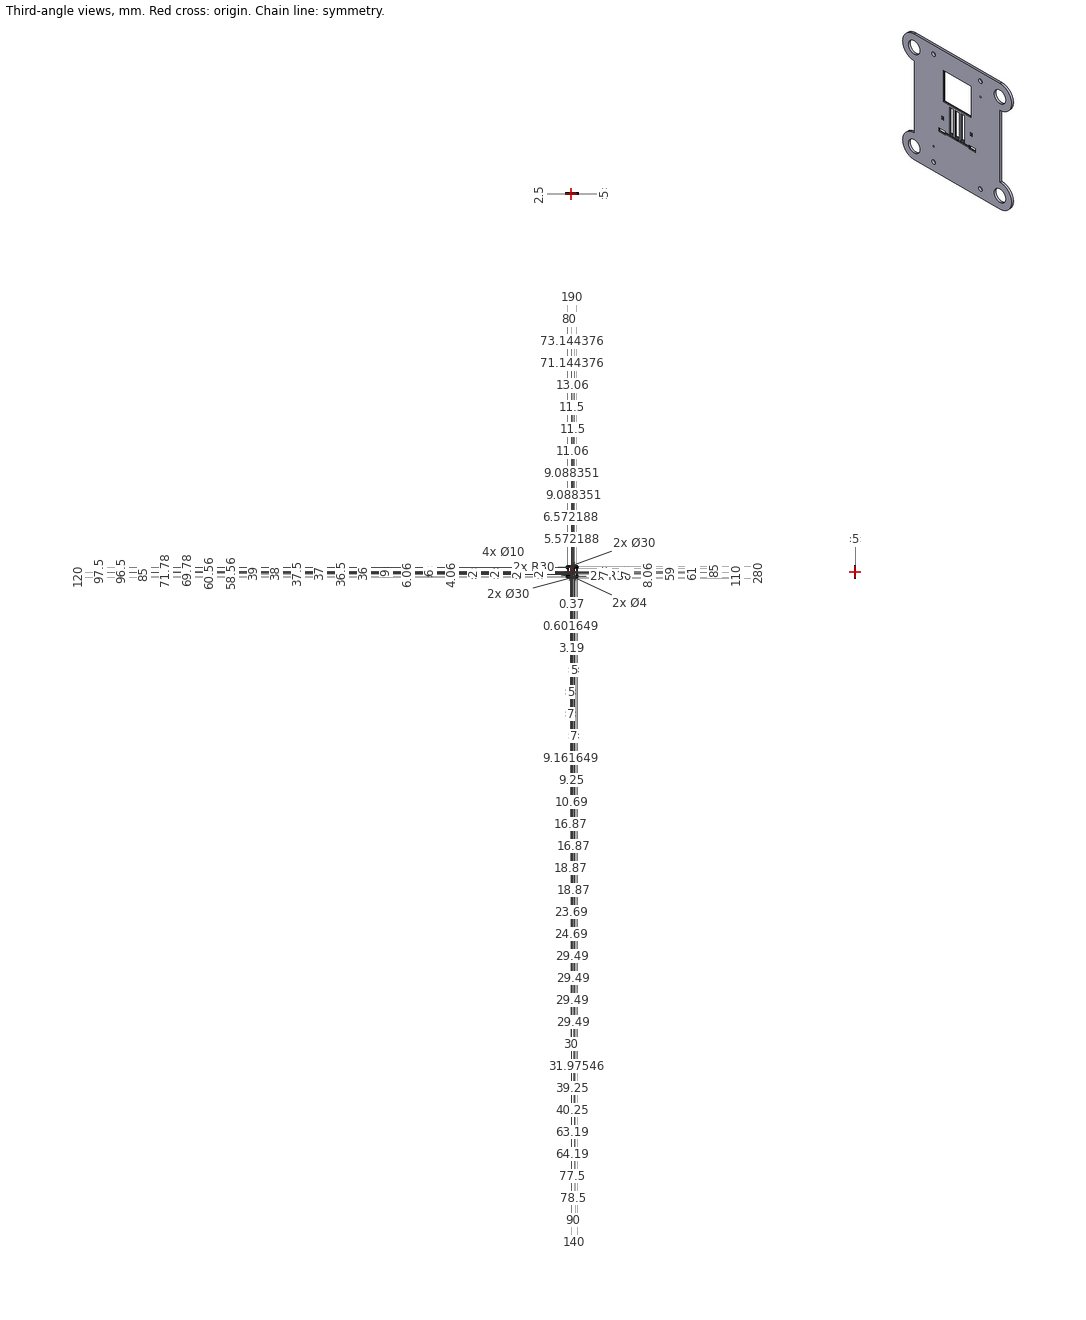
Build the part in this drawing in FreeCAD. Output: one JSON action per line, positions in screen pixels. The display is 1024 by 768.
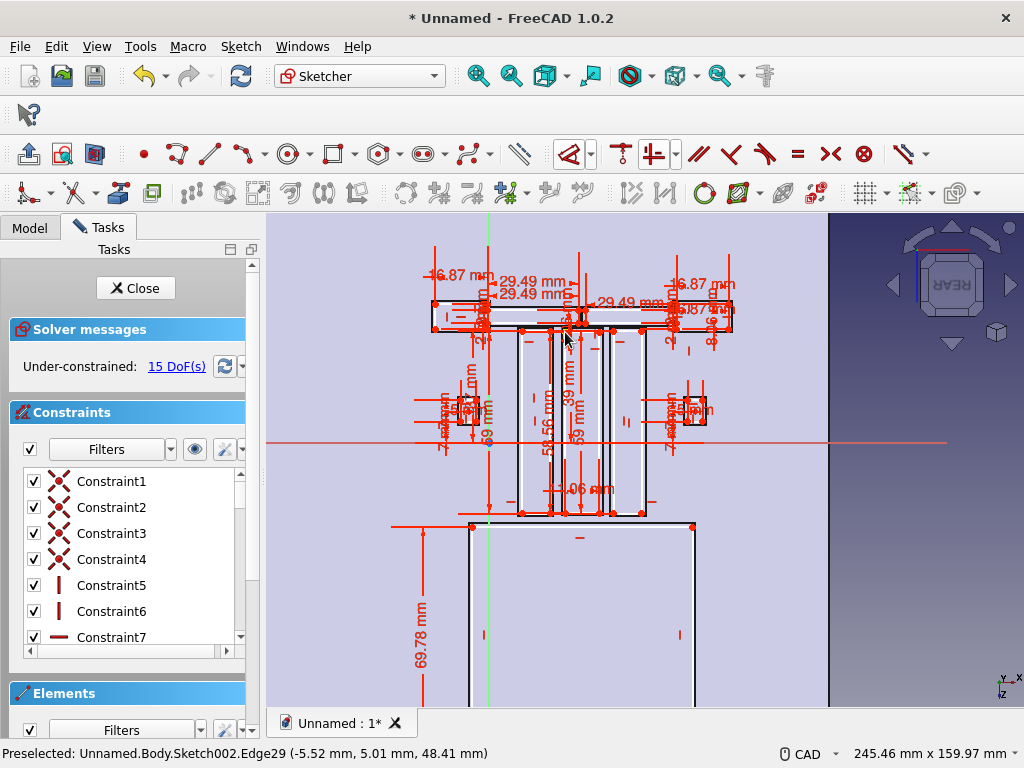
{"action": "left_click", "coordinate": [565, 332]}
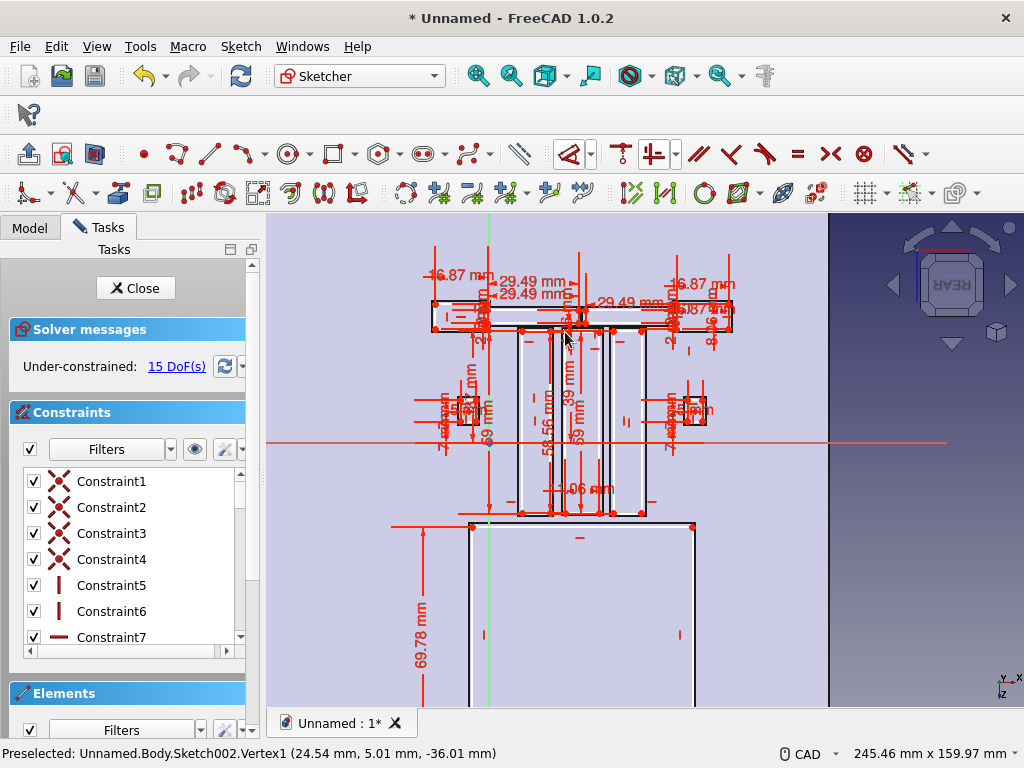
{"action": "key", "text": "i"}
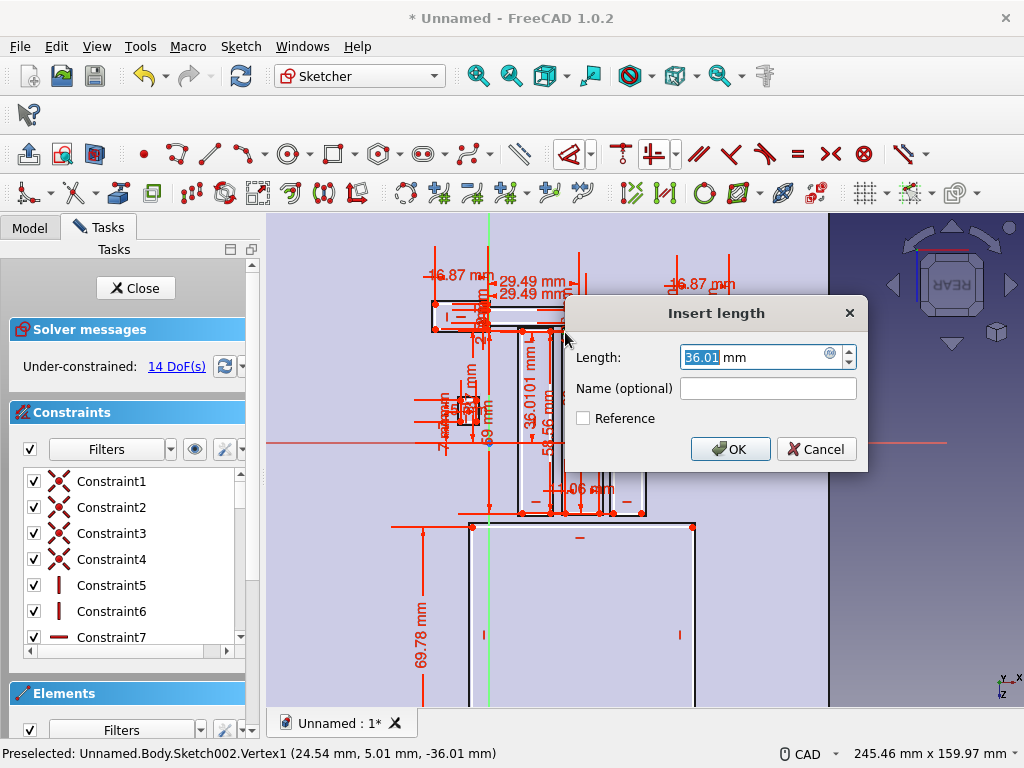
{"action": "type", "text": "36.5"}
{"action": "key", "text": "Return"}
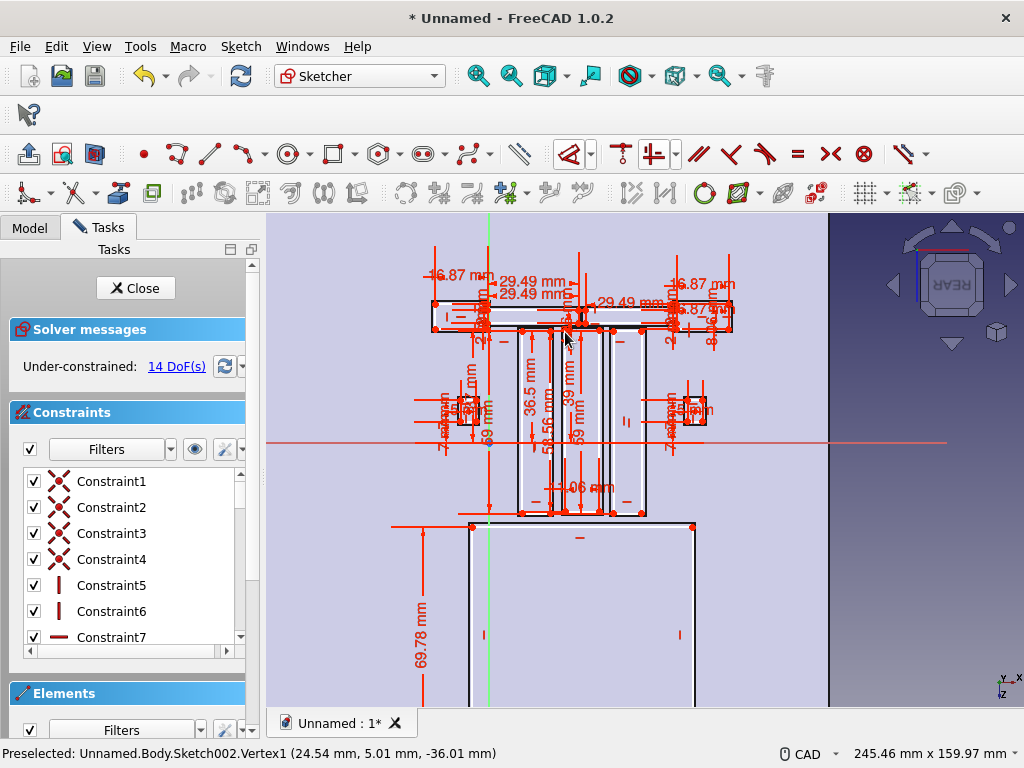
{"action": "left_click", "coordinate": [729, 329]}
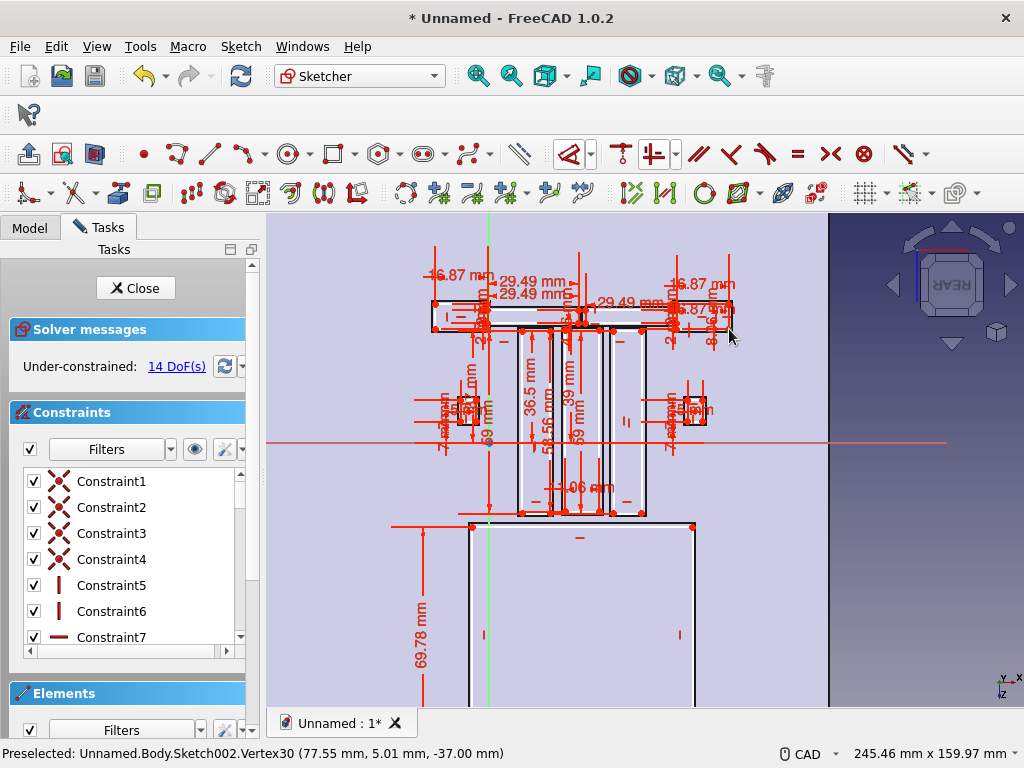
{"action": "left_click", "coordinate": [590, 154]}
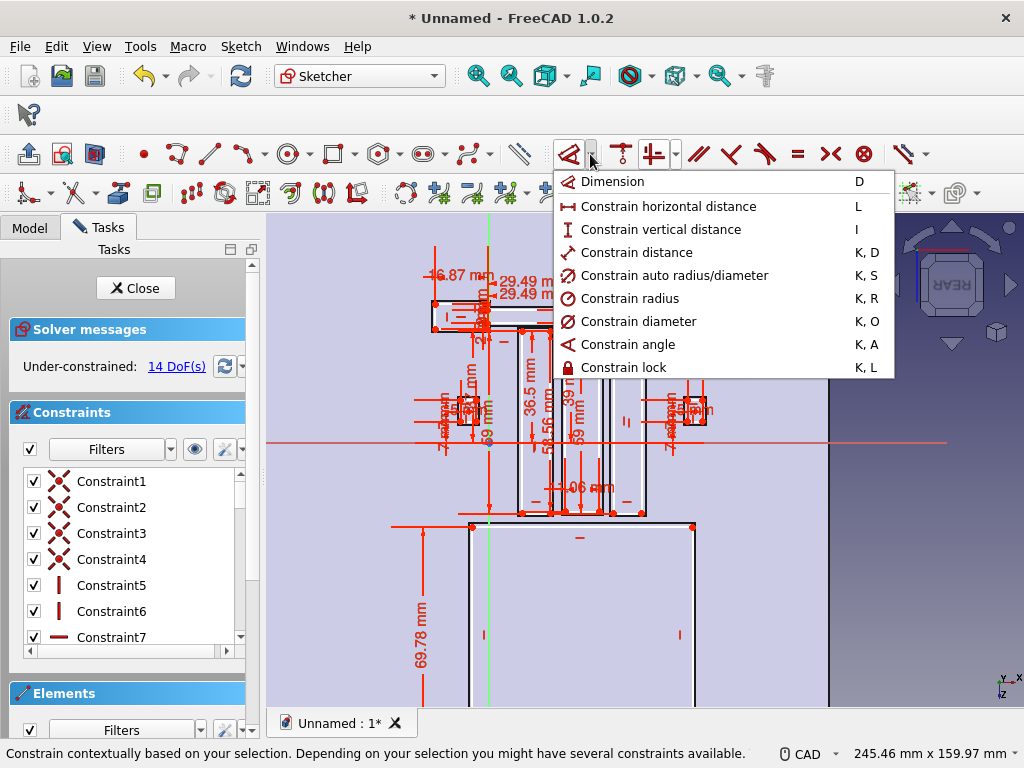
{"action": "left_click", "coordinate": [724, 206]}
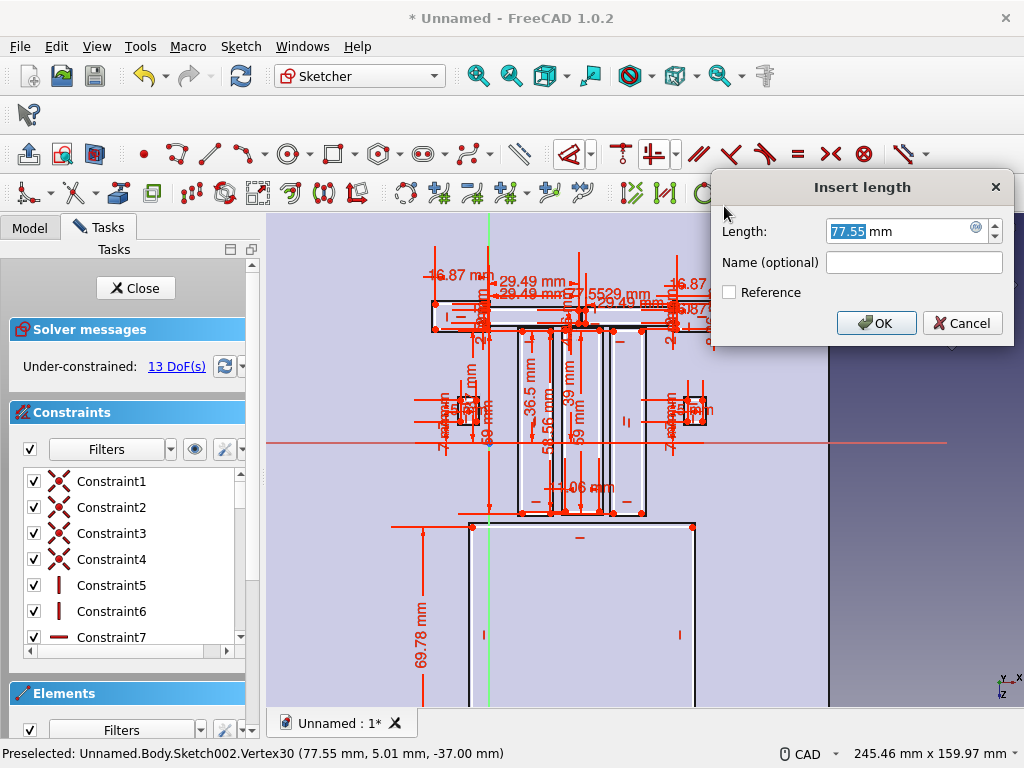
{"action": "type", "text": "77.5"}
{"action": "key", "text": "Return"}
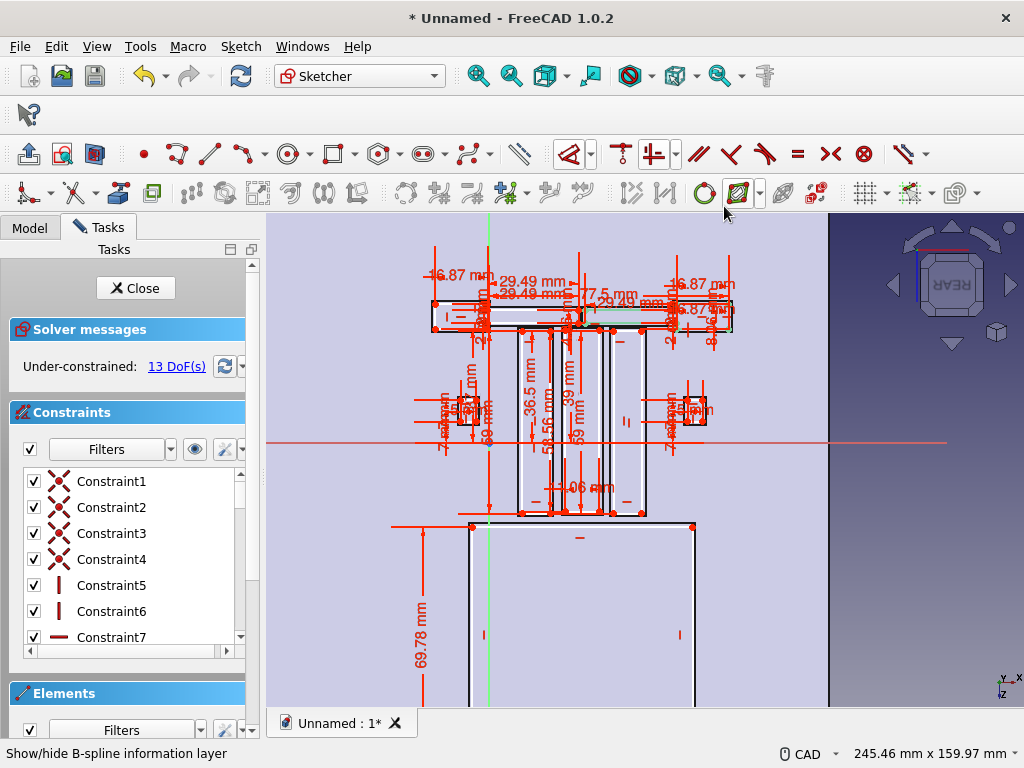
{"action": "left_click", "coordinate": [614, 331]}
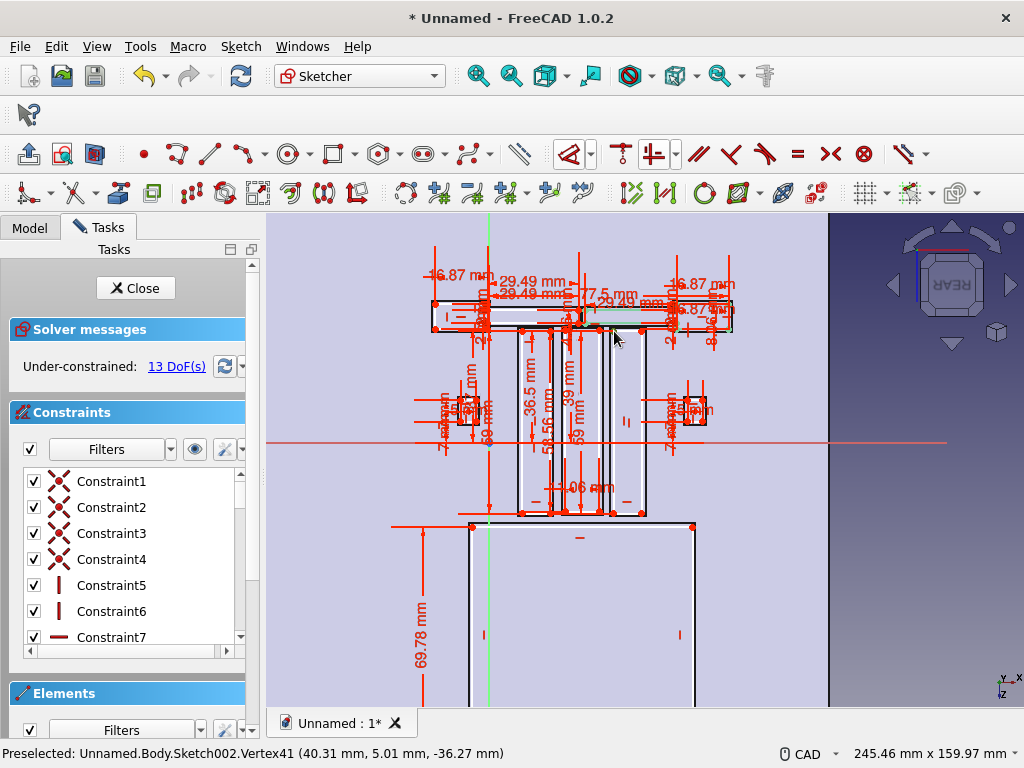
{"action": "left_click", "coordinate": [590, 154]}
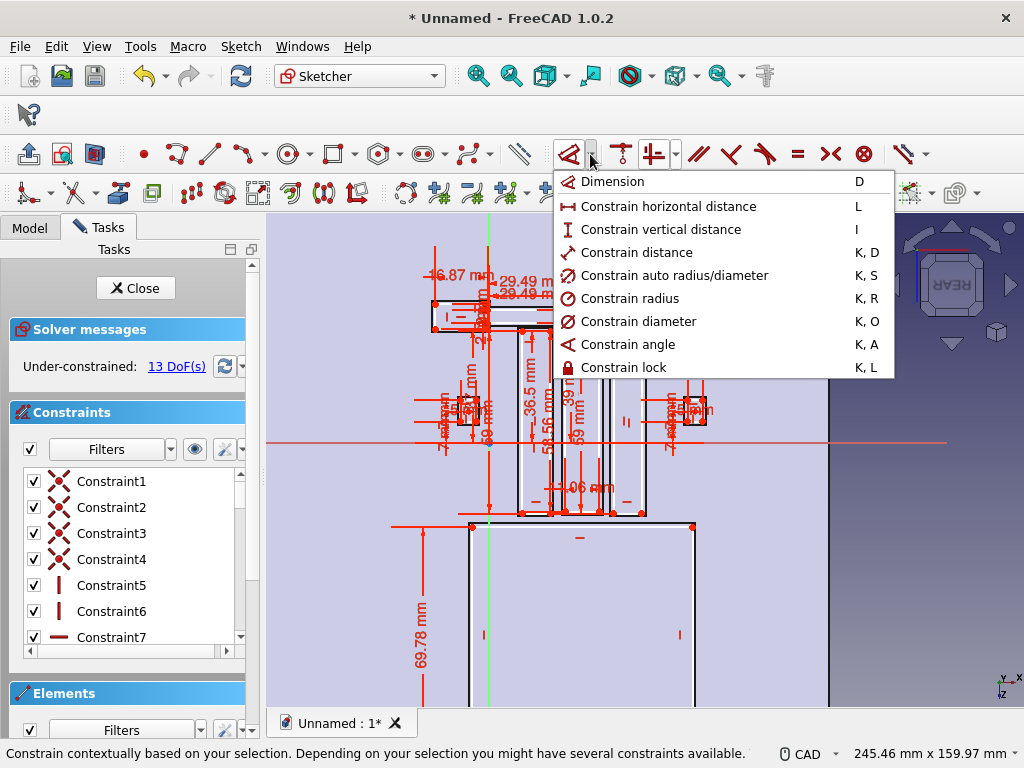
{"action": "left_click", "coordinate": [724, 230]}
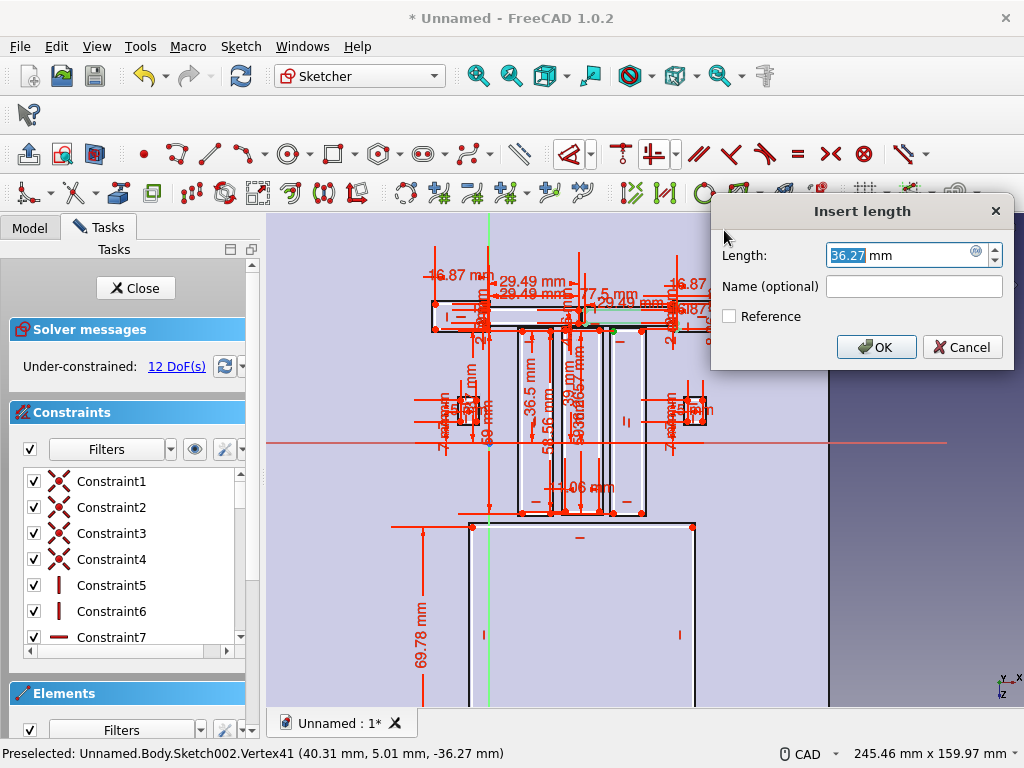
{"action": "type", "text": "36.5"}
{"action": "key", "text": "Return"}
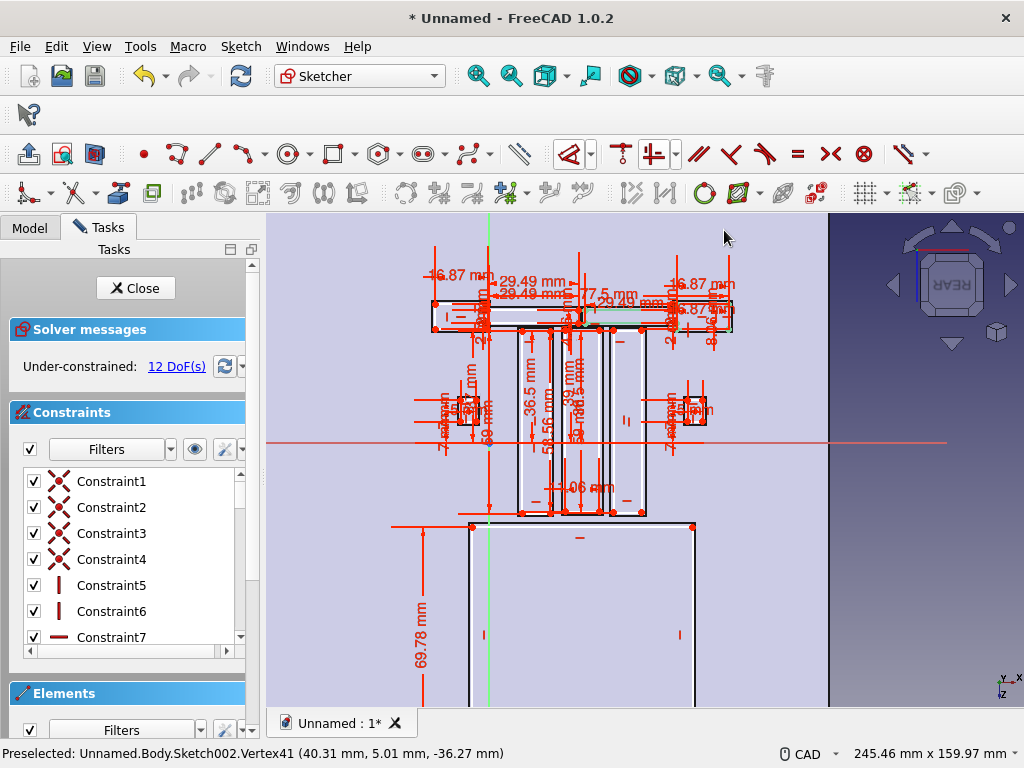
{"action": "scroll", "coordinate": [565, 332], "scroll_direction": "down", "scroll_amount": 2}